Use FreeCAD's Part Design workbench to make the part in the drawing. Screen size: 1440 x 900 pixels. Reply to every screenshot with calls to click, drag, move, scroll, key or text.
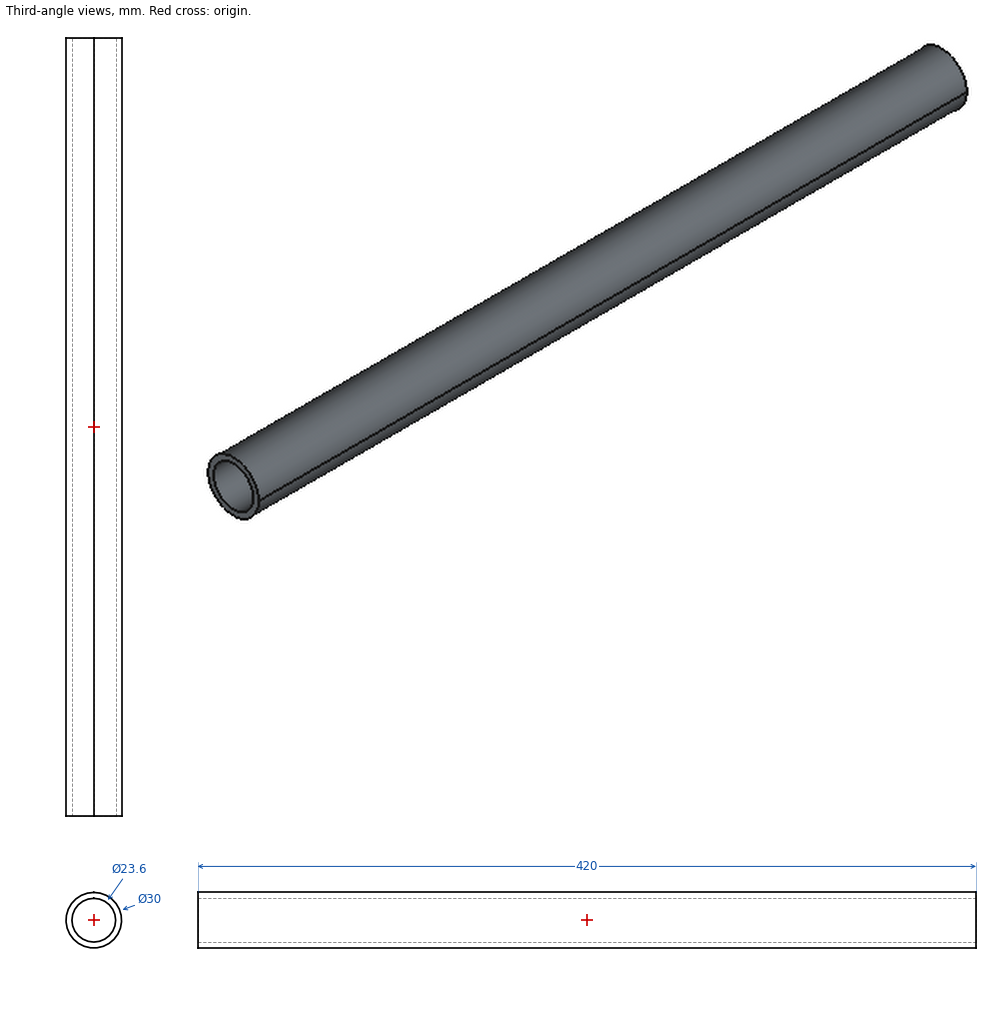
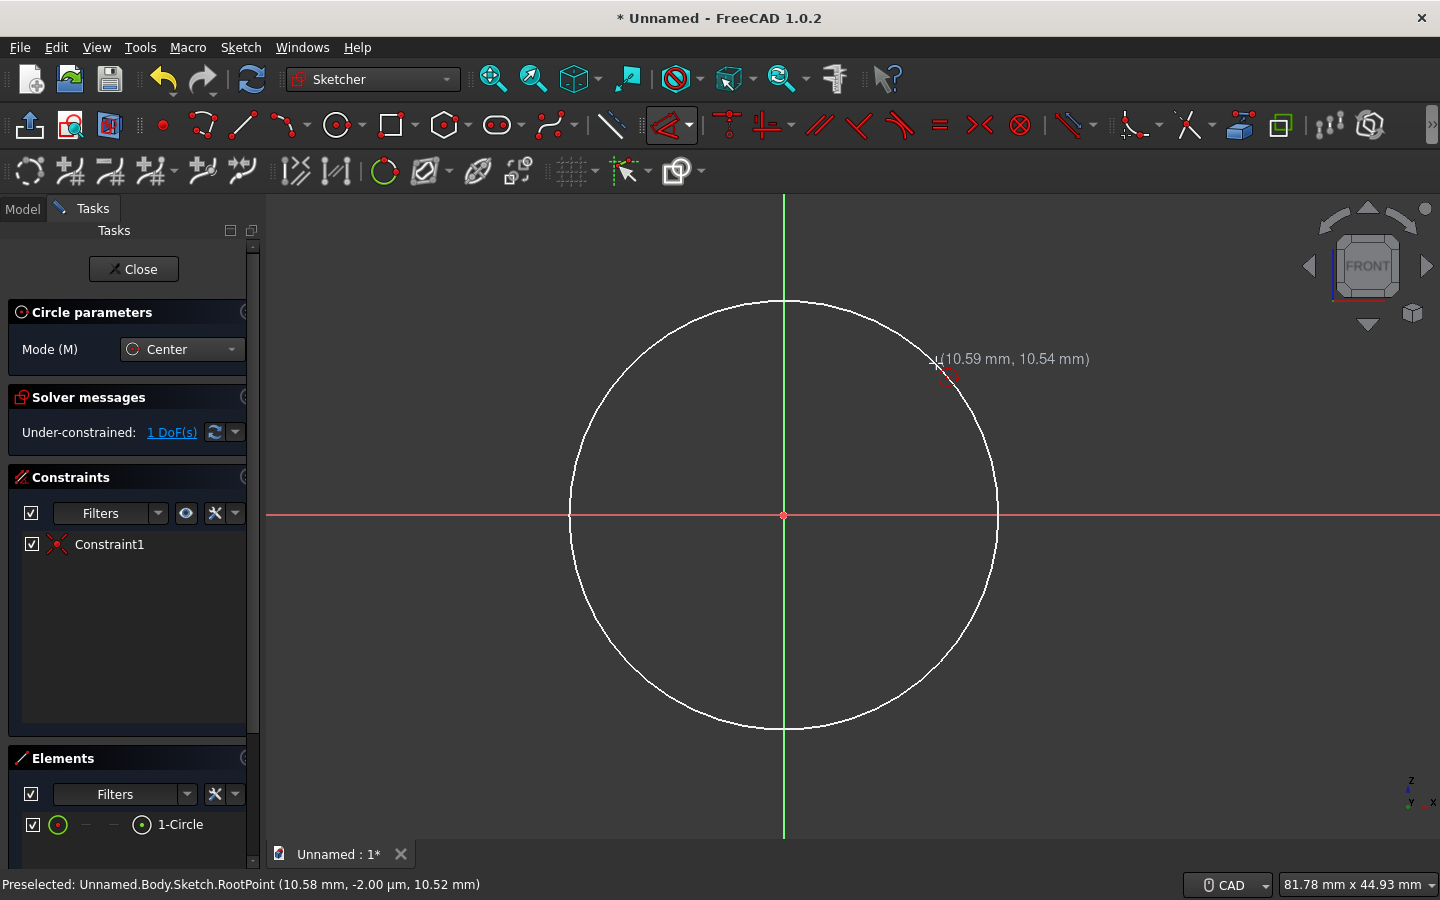
click(784, 515)
click(904, 396)
key(Escape)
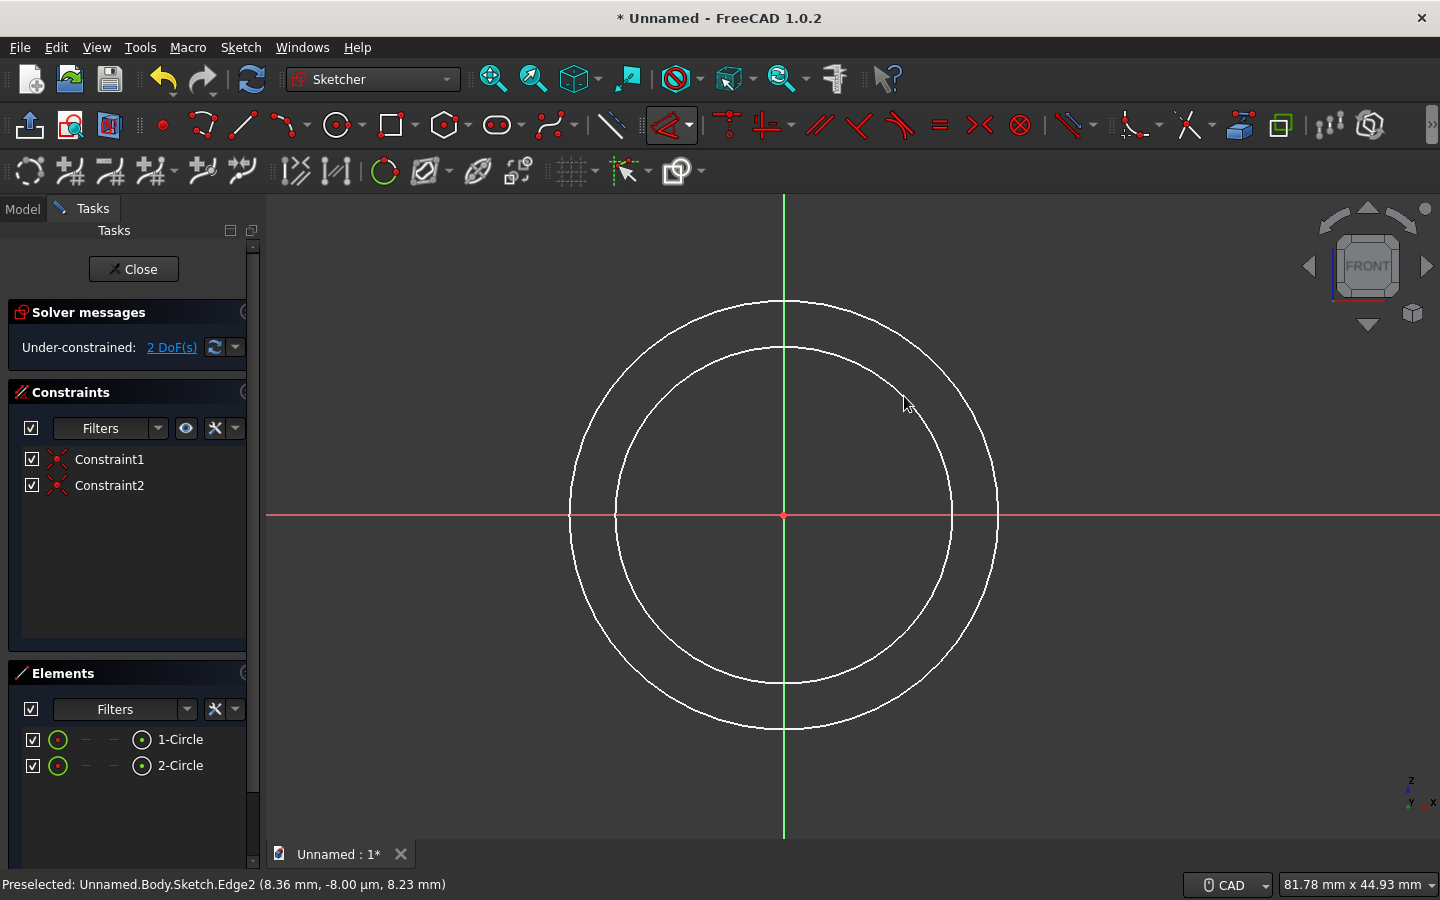
click(666, 126)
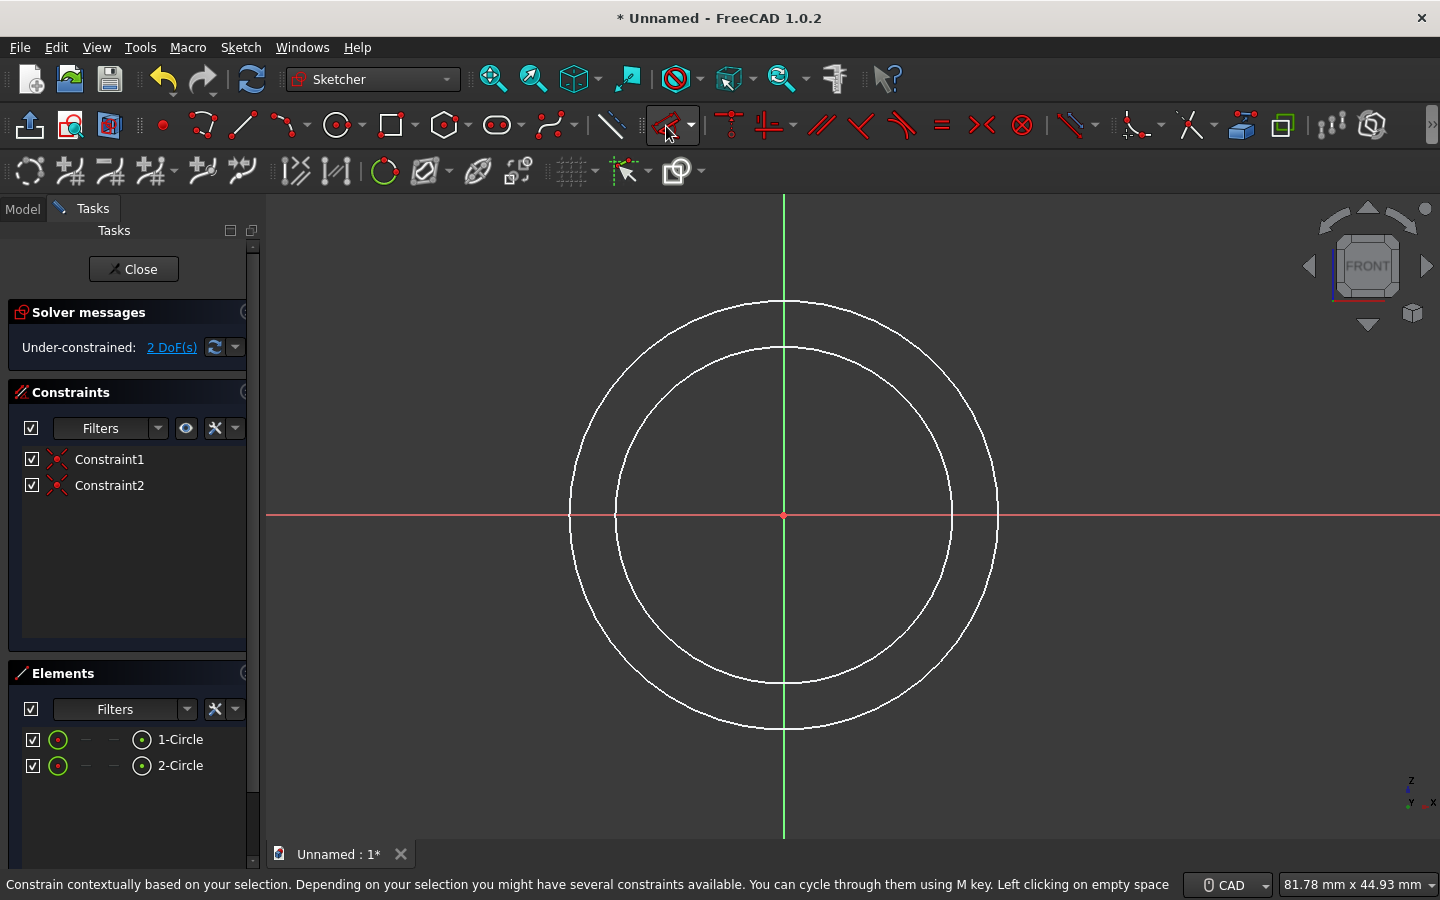
click(935, 363)
click(958, 340)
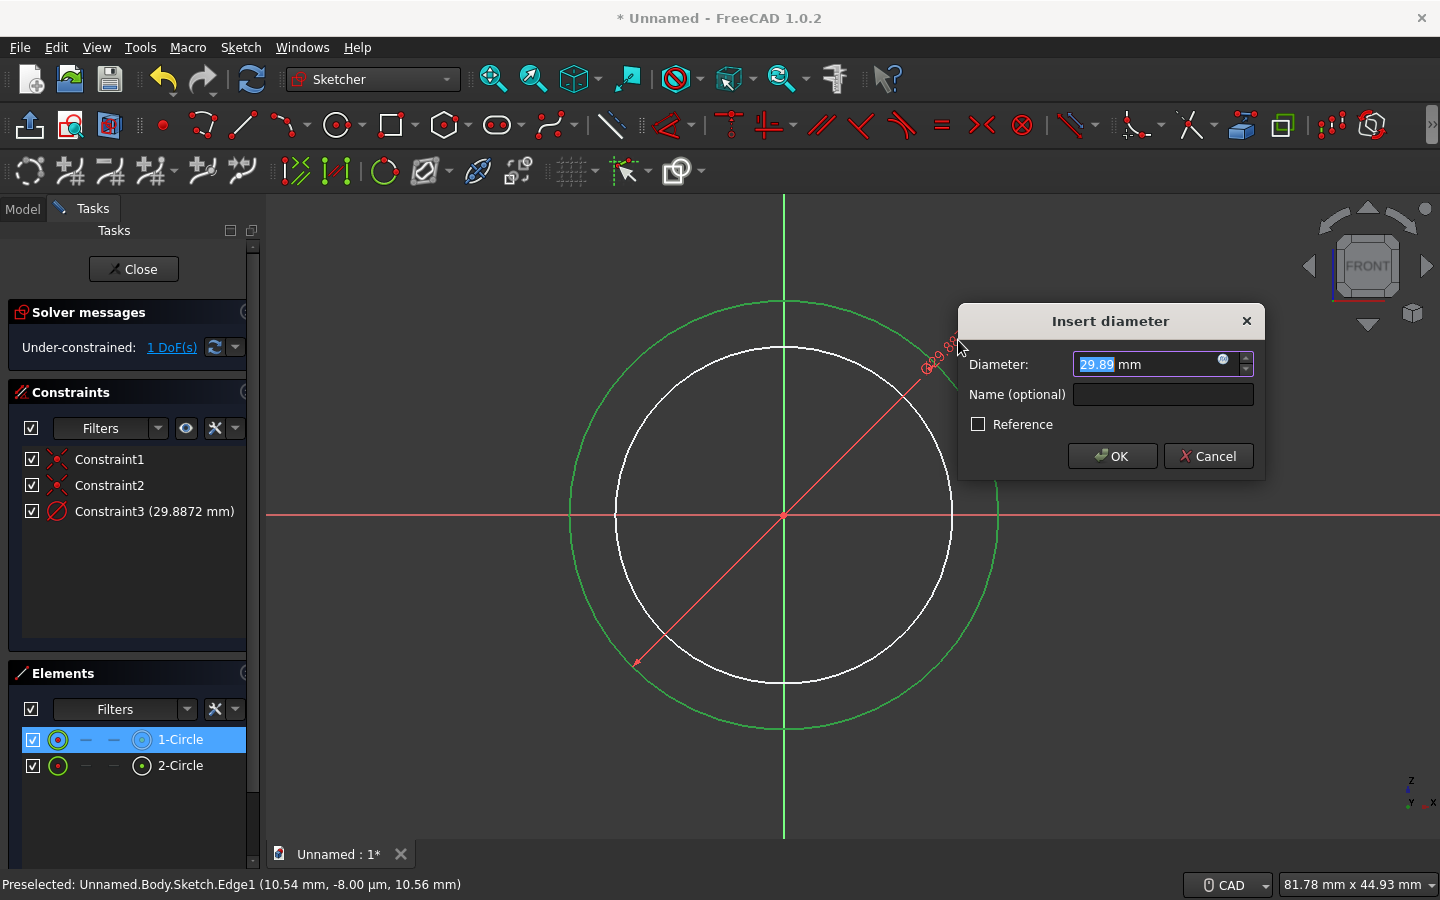
text(30)
key(Return)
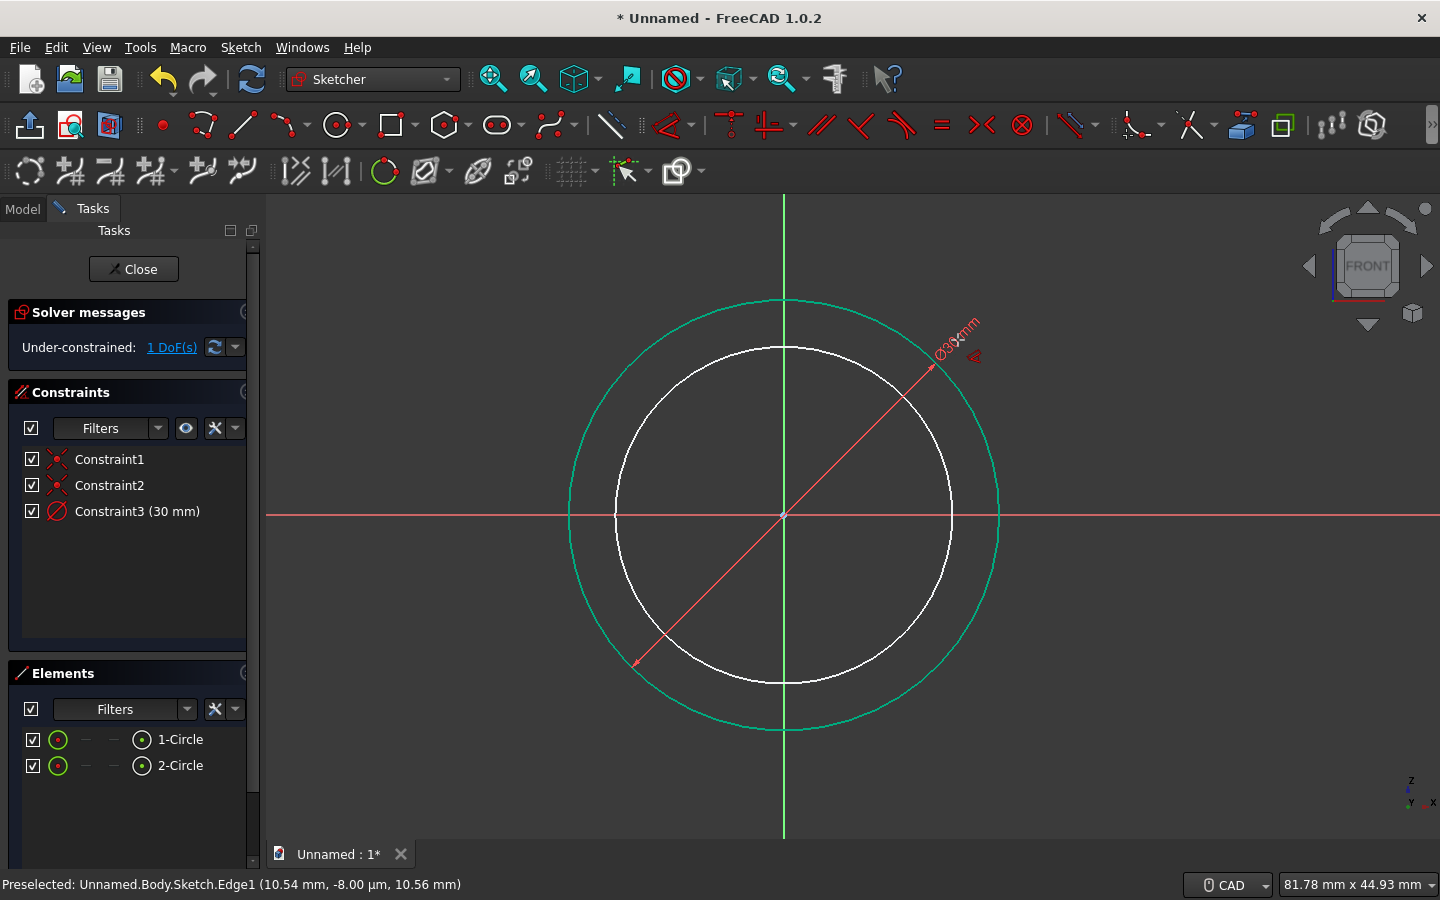
click(903, 396)
click(926, 373)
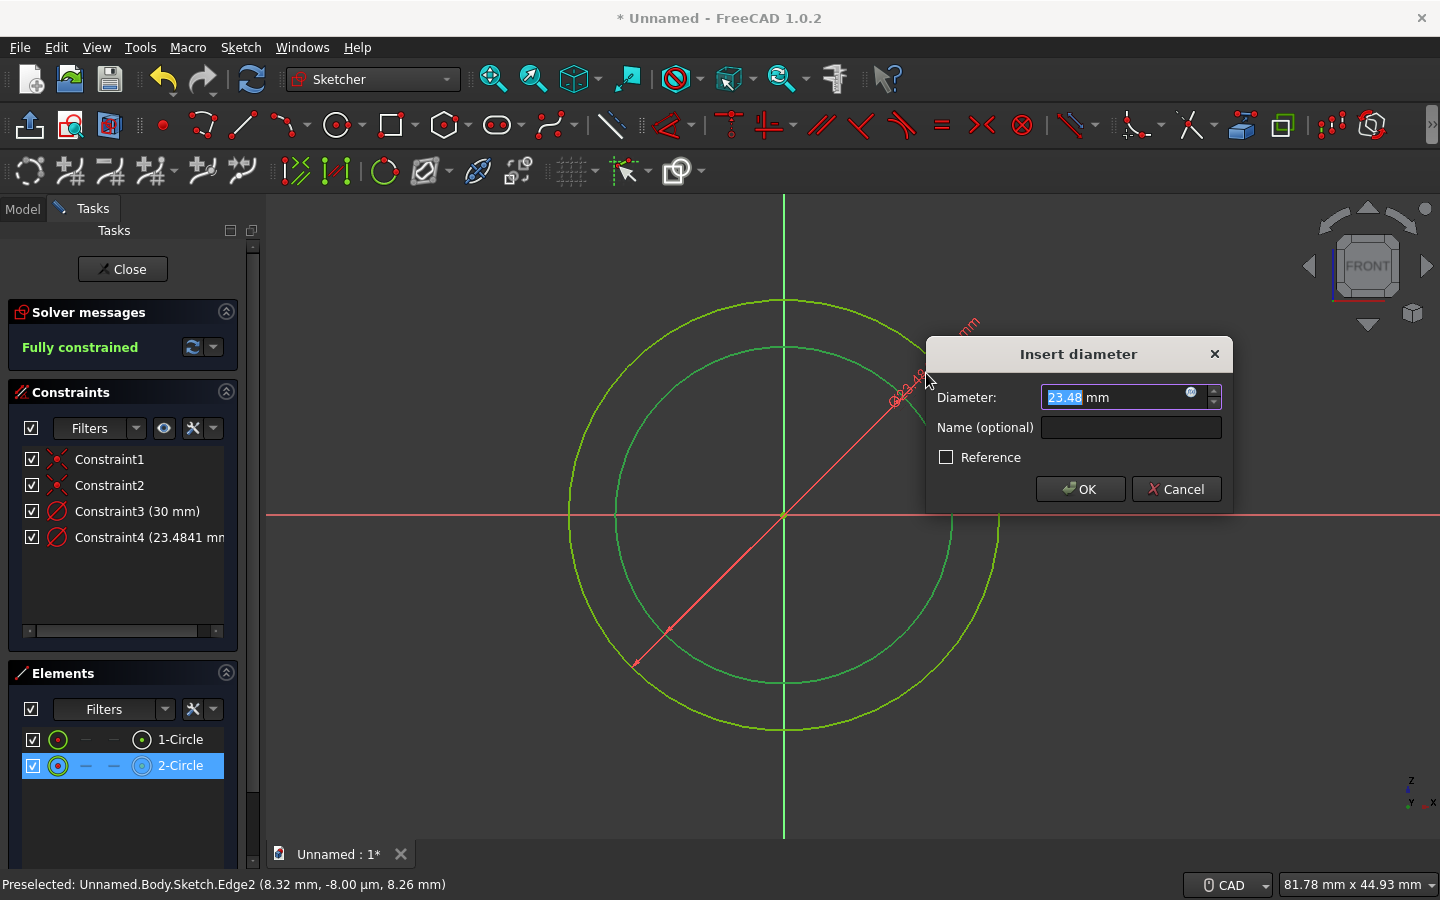
text(23.6)
key(Return)
key(Escape)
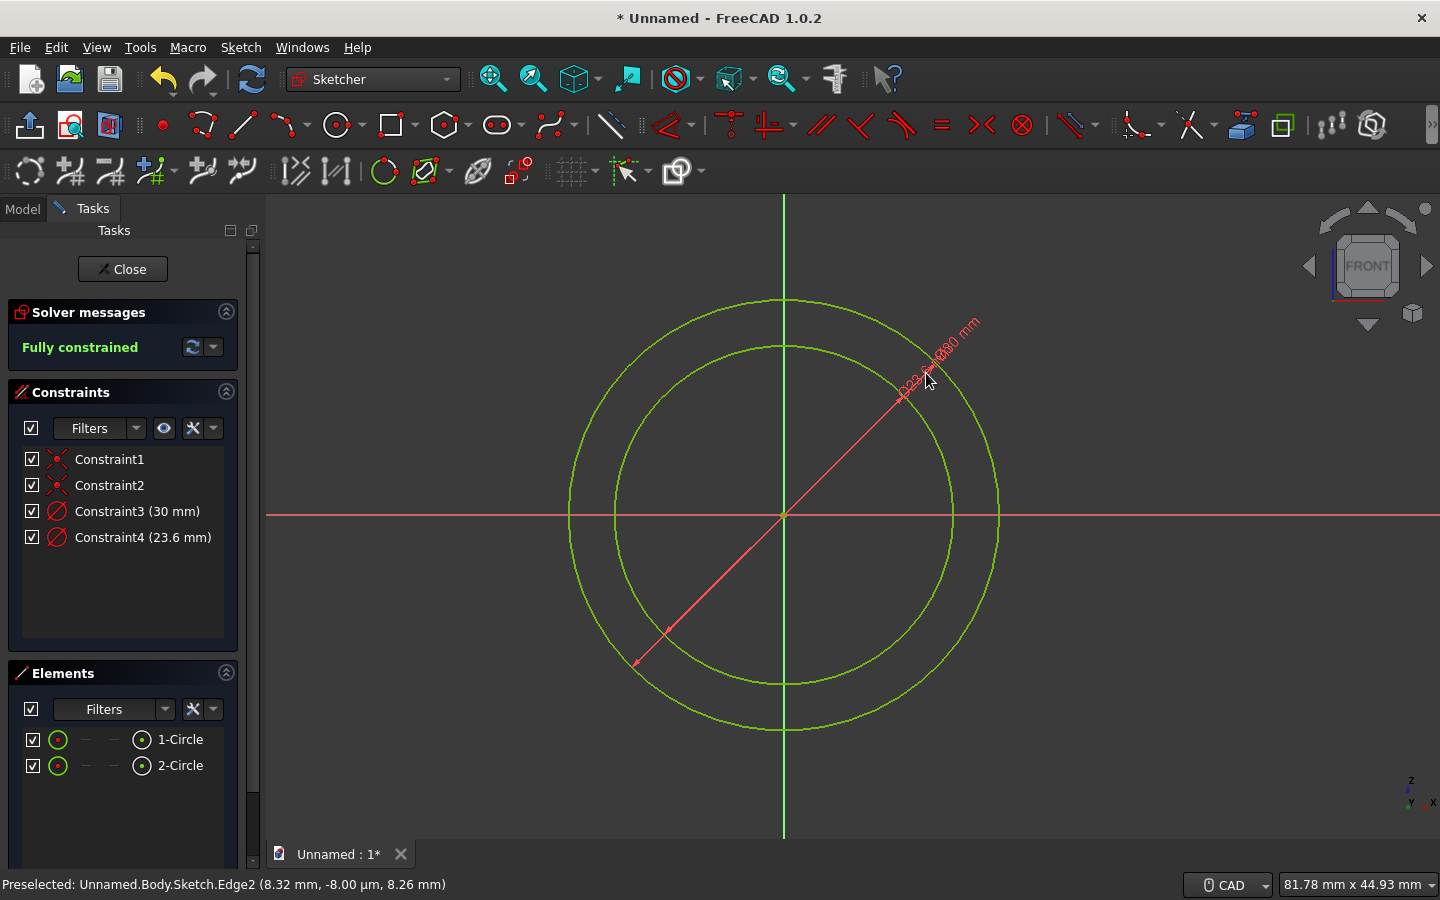
click(123, 269)